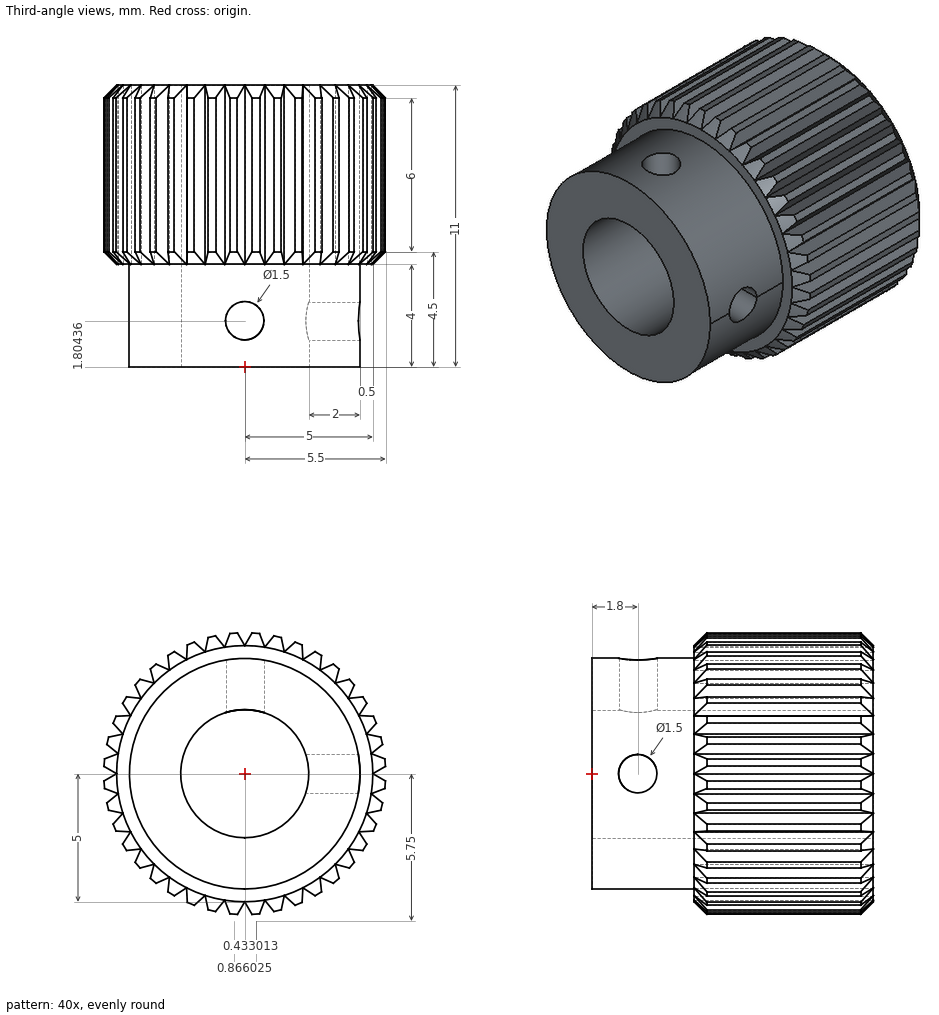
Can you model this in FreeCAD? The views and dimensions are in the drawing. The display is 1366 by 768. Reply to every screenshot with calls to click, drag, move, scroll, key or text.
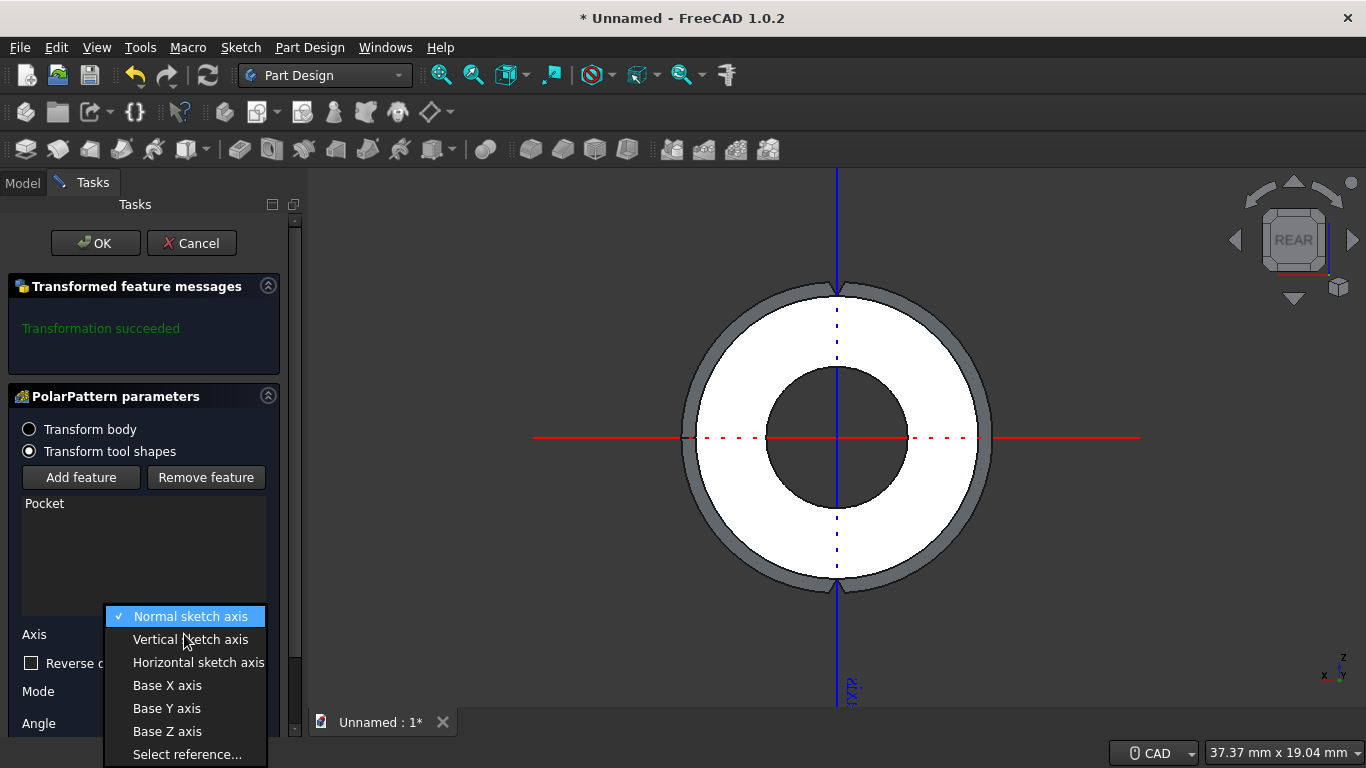
click(184, 708)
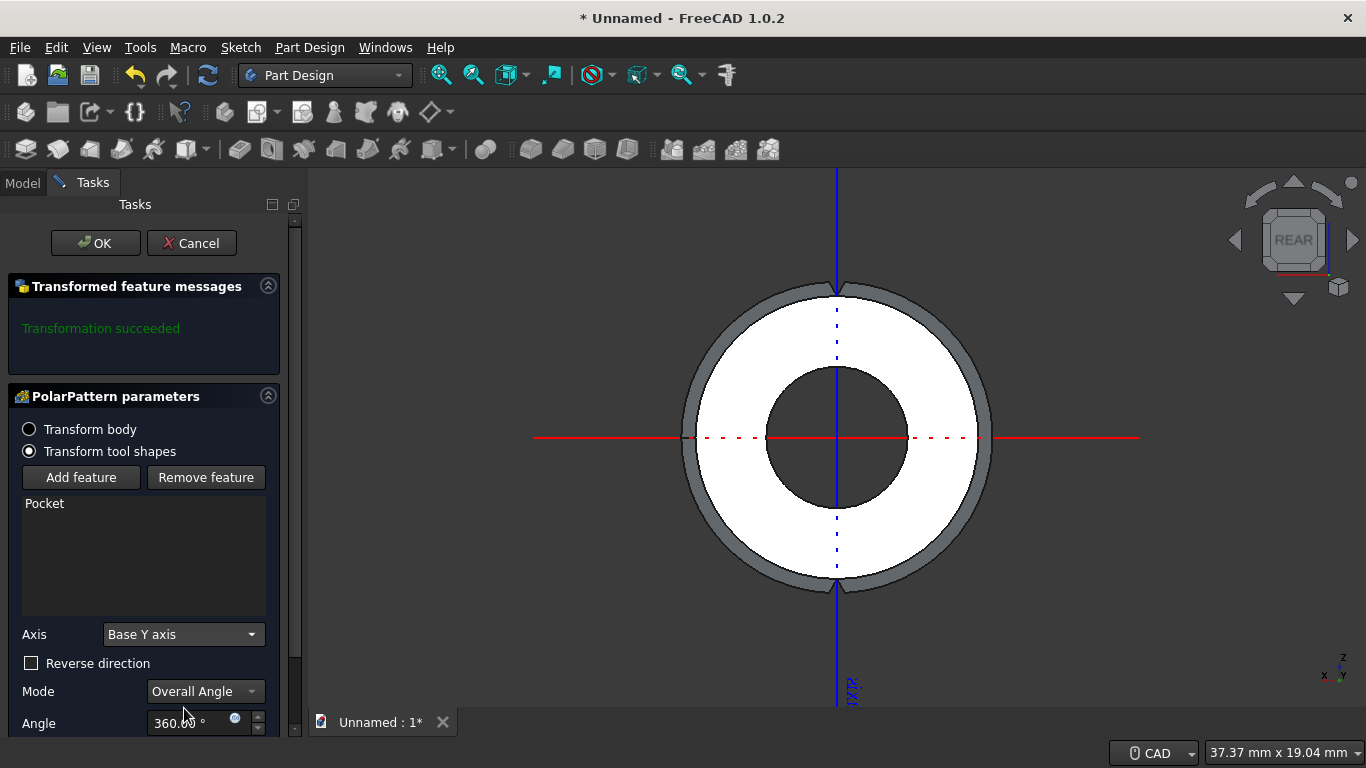
scroll(295, 475, down, 2)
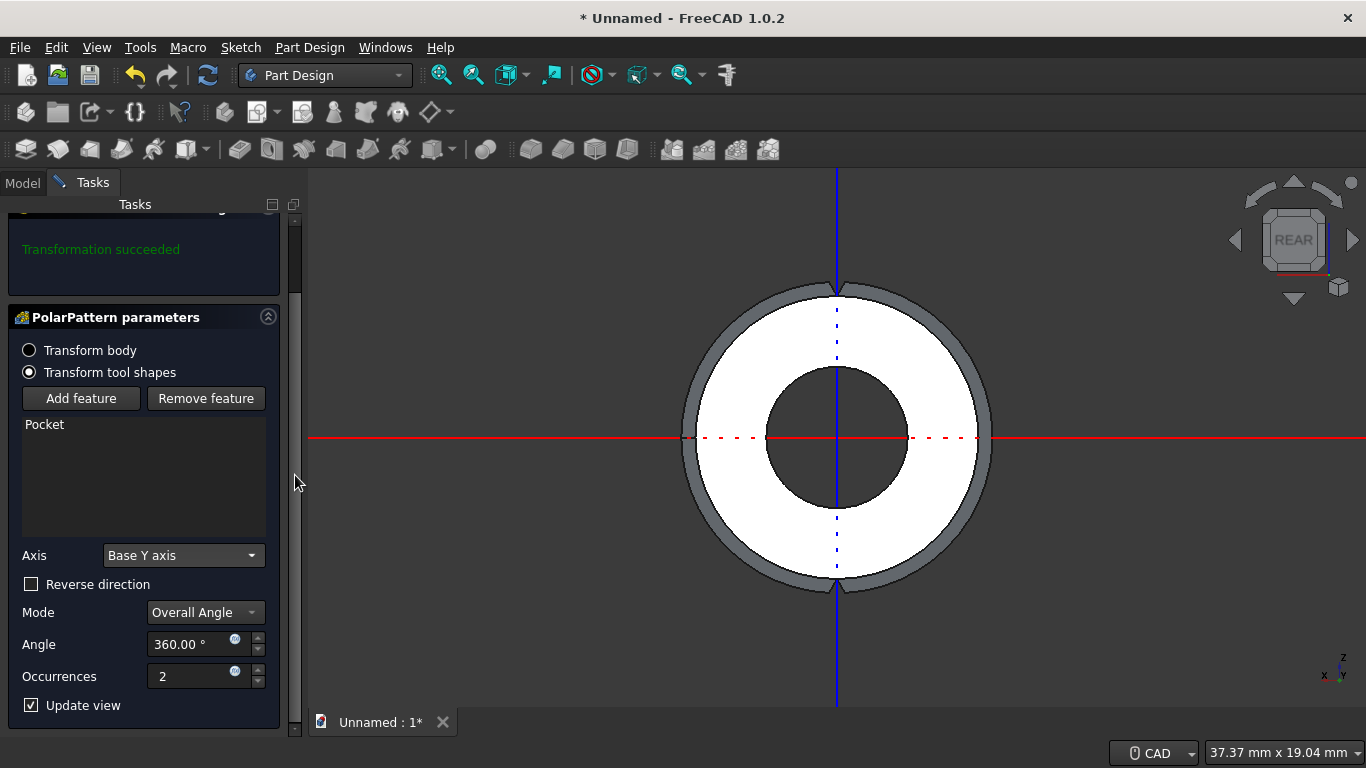
triple_click(198, 676)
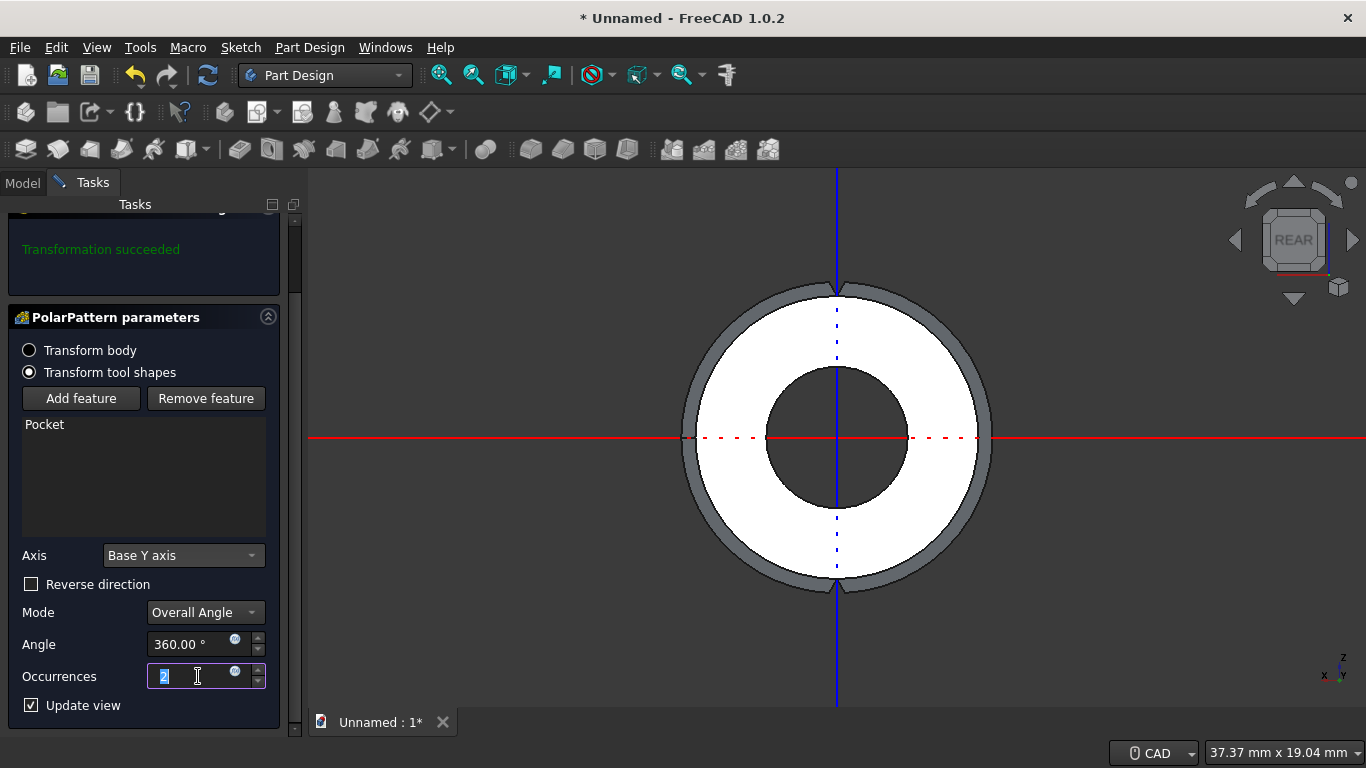
text(40)
key(Tab)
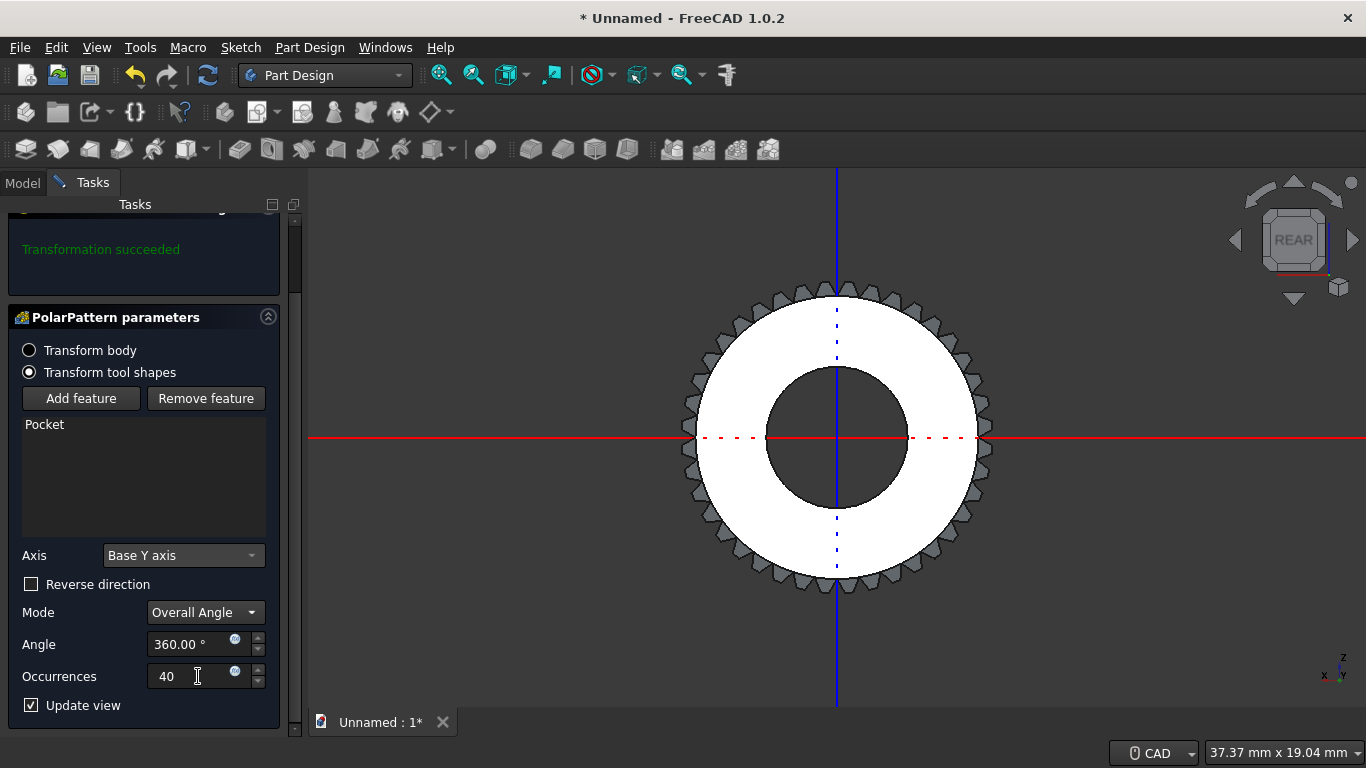
scroll(295, 475, up, 3)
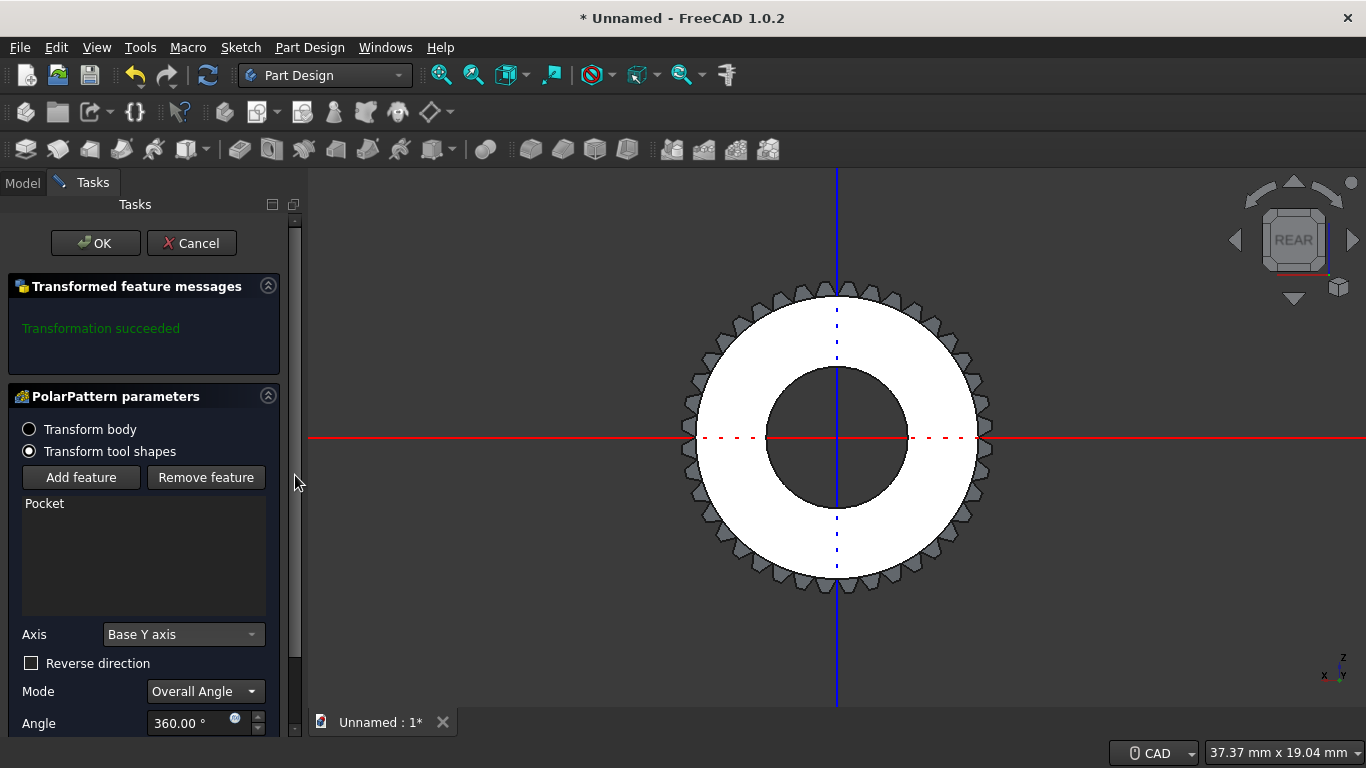
click(96, 243)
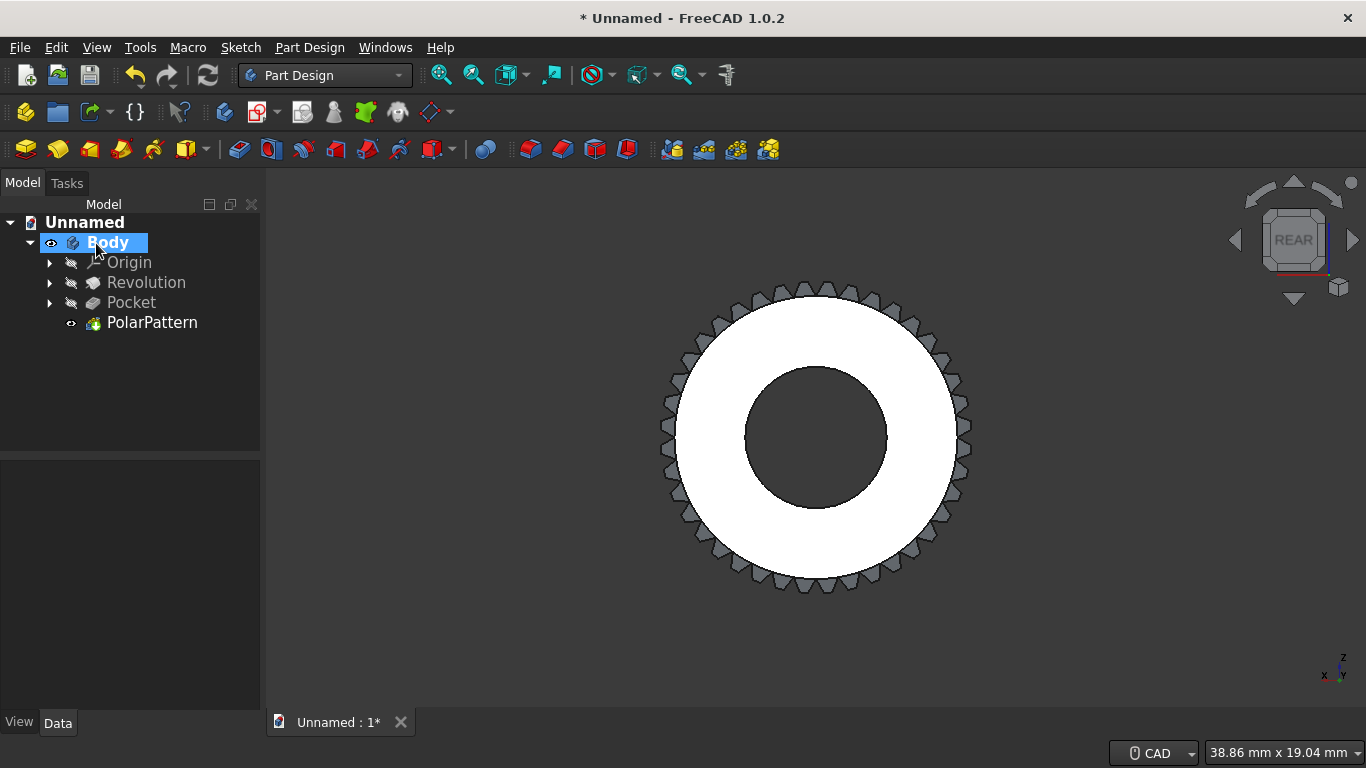
click(258, 112)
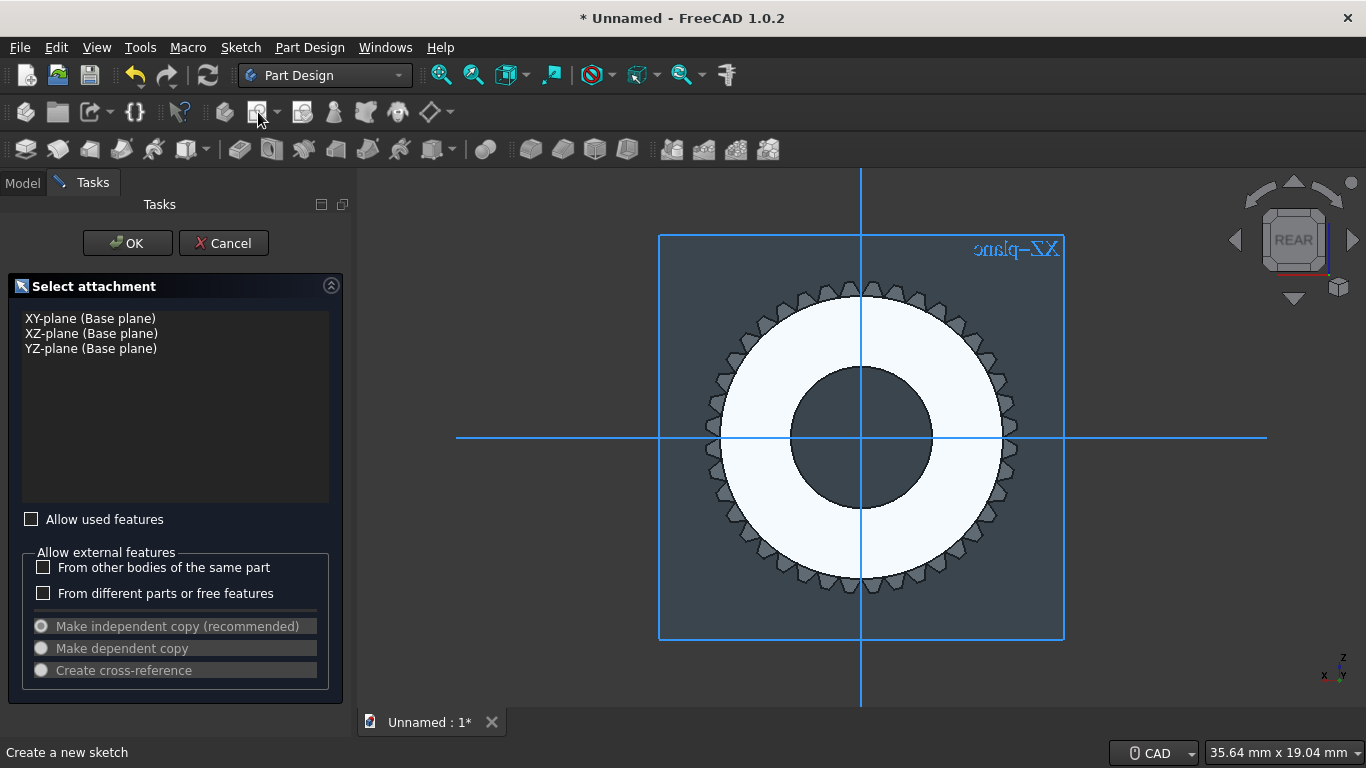
click(82, 318)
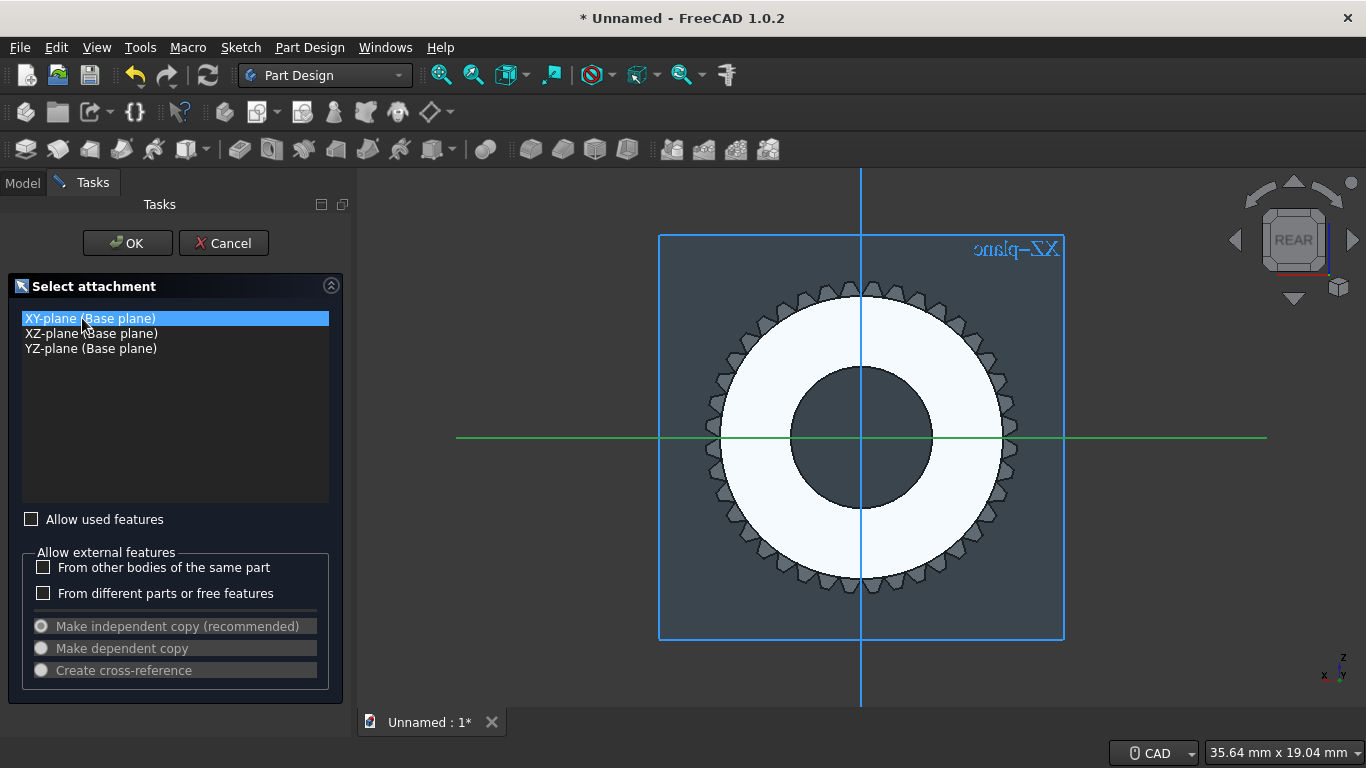
click(128, 243)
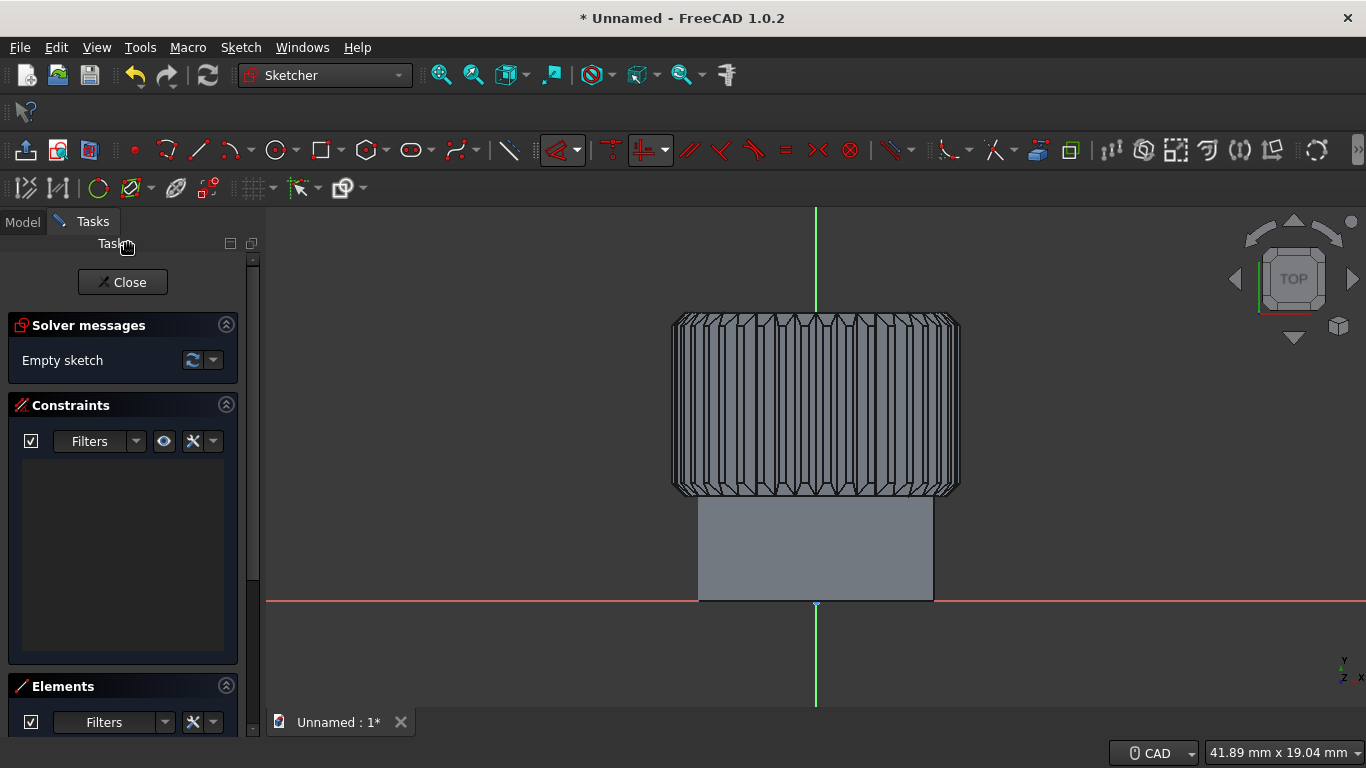
click(90, 150)